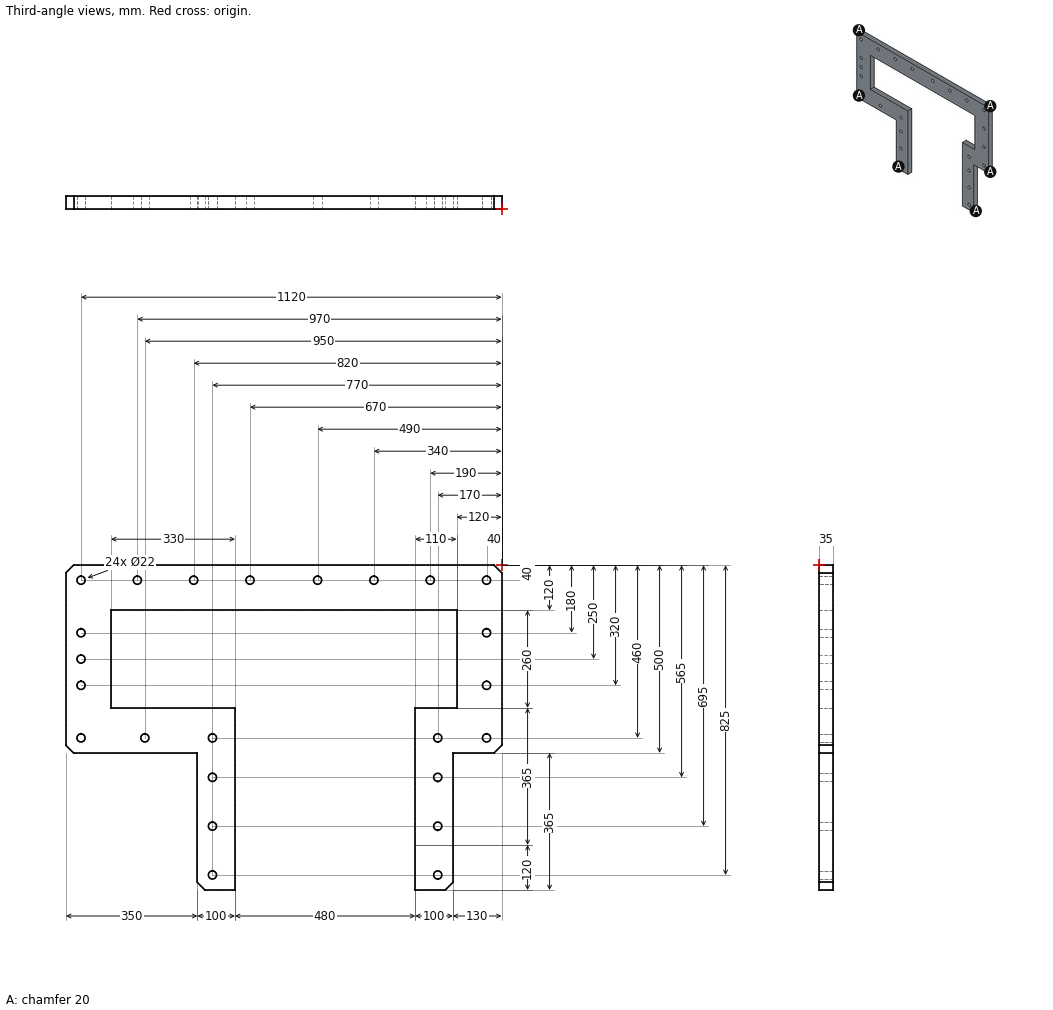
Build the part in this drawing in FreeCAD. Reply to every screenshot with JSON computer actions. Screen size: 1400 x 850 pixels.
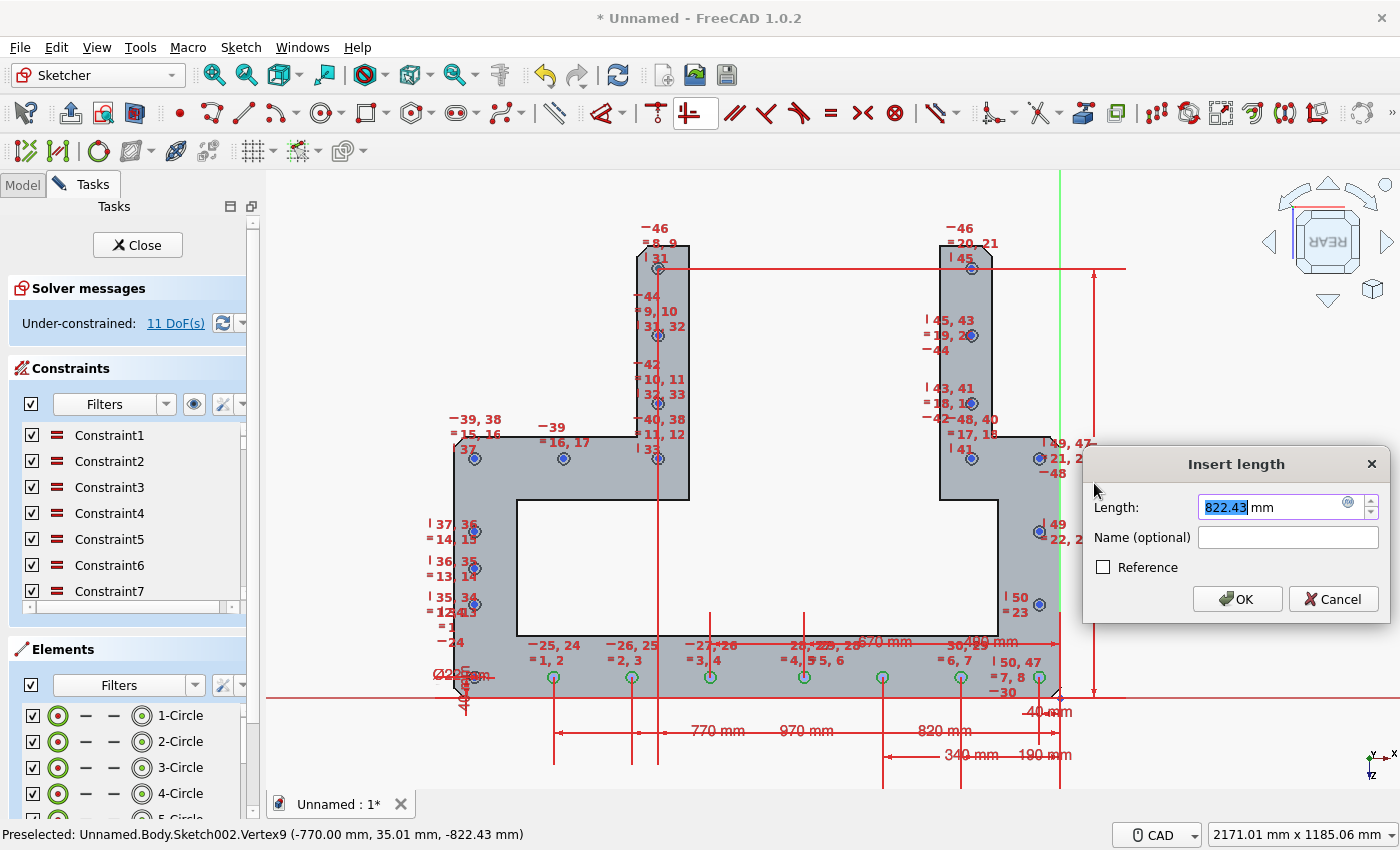
{"action": "type", "text": "825"}
{"action": "key", "text": "Return"}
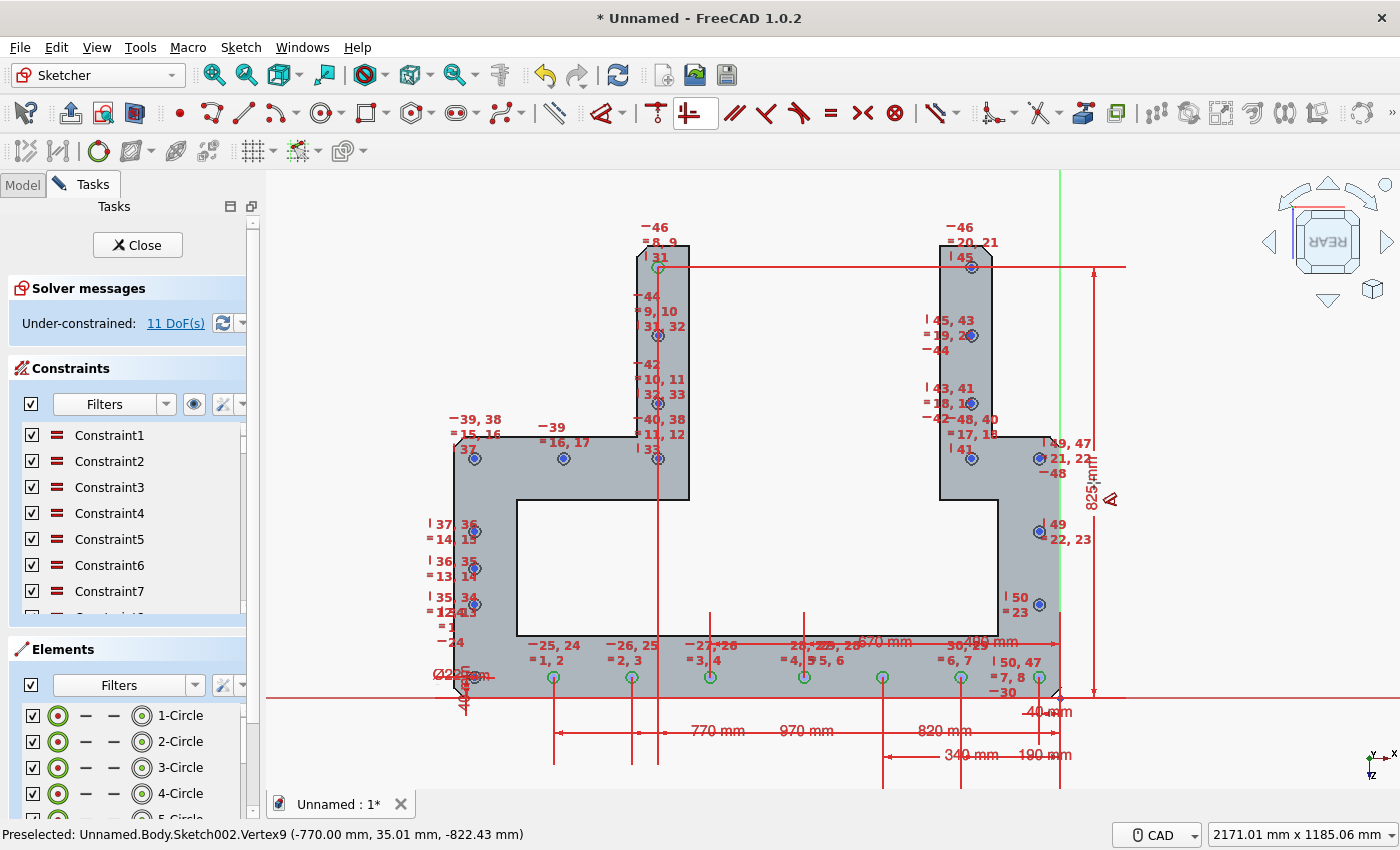
{"action": "left_click", "coordinate": [658, 336]}
{"action": "left_click", "coordinate": [1094, 517]}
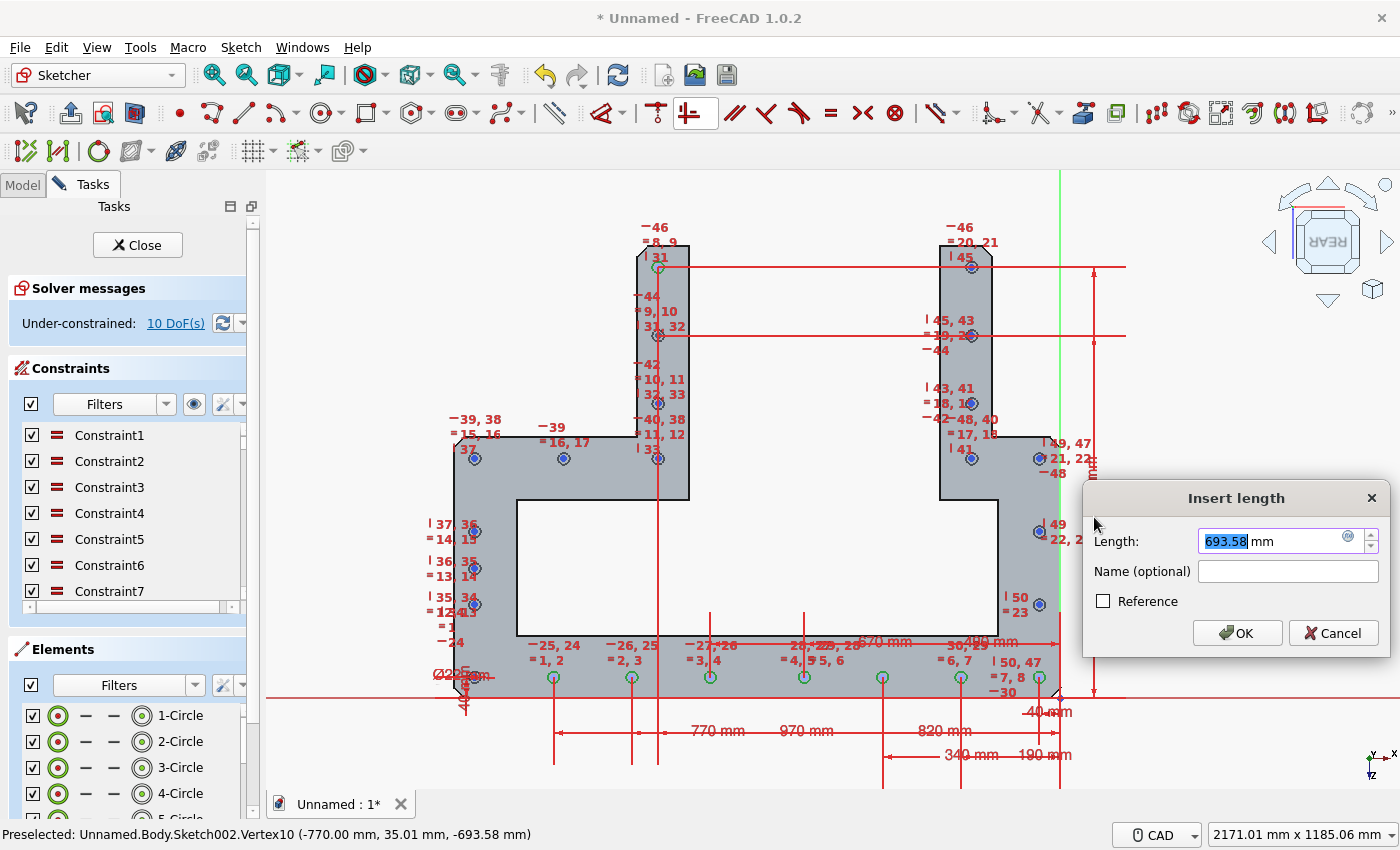
{"action": "type", "text": "695"}
{"action": "key", "text": "Return"}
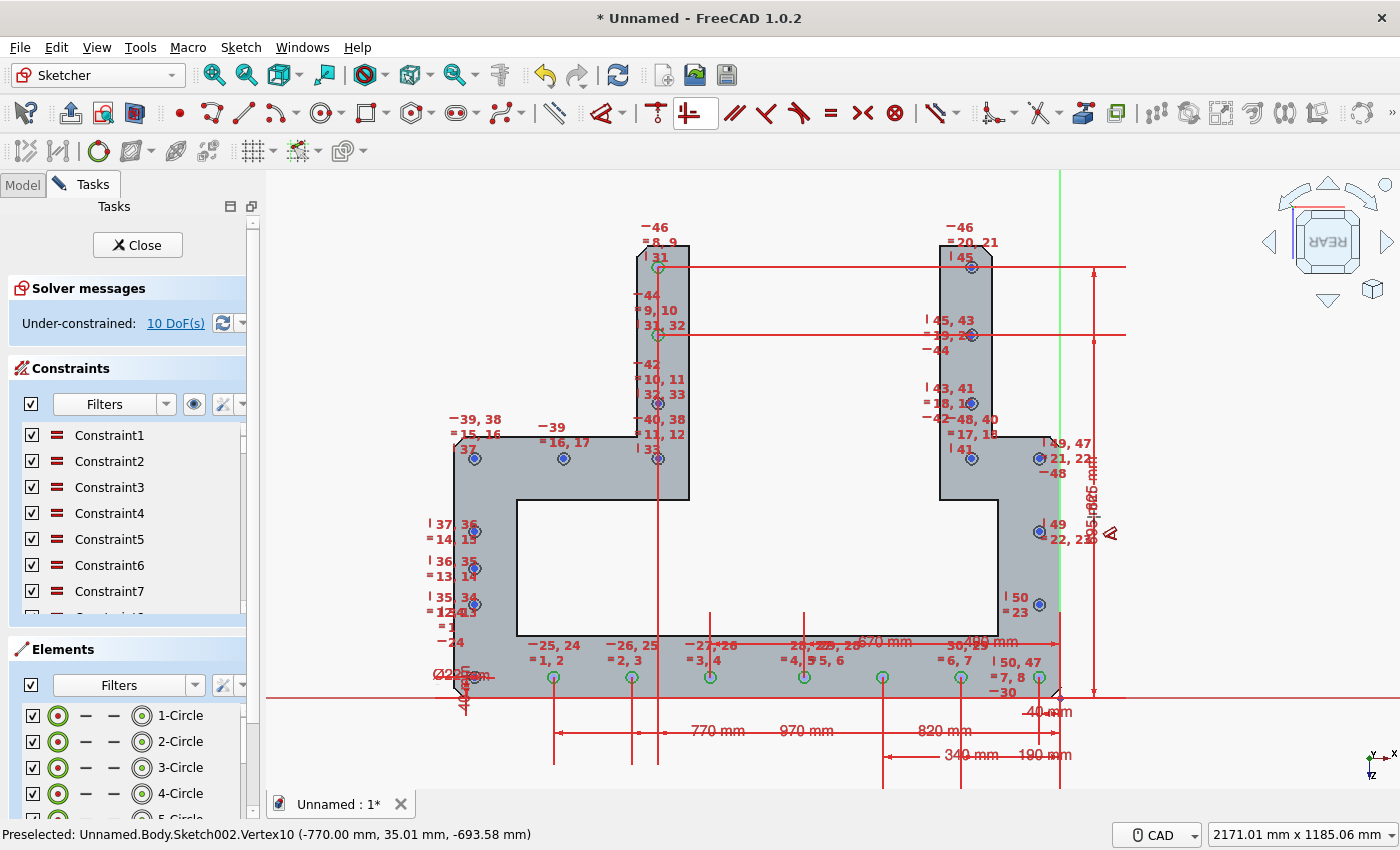
{"action": "left_click", "coordinate": [658, 404]}
{"action": "left_click", "coordinate": [1094, 551]}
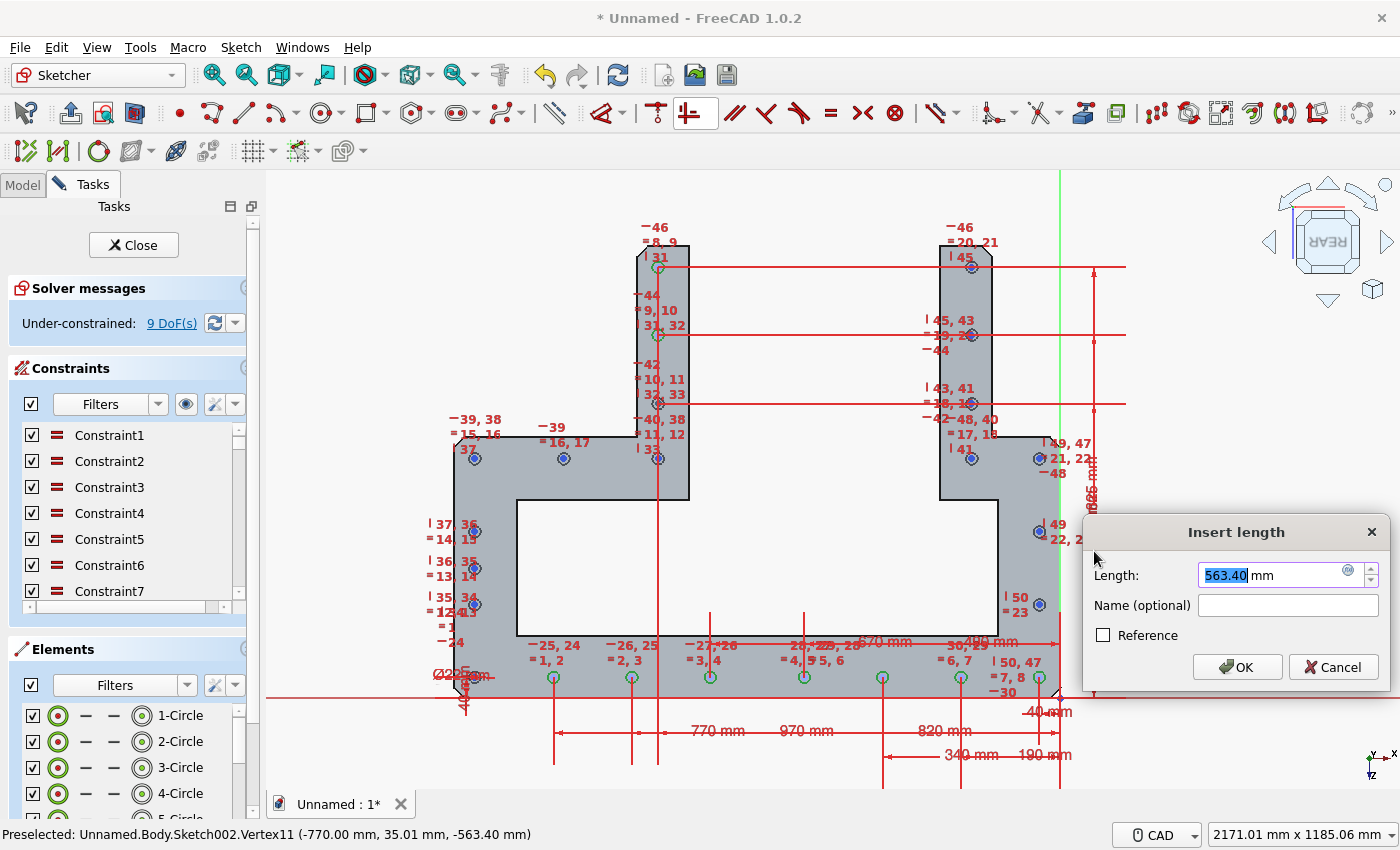
{"action": "type", "text": "565"}
{"action": "key", "text": "Return"}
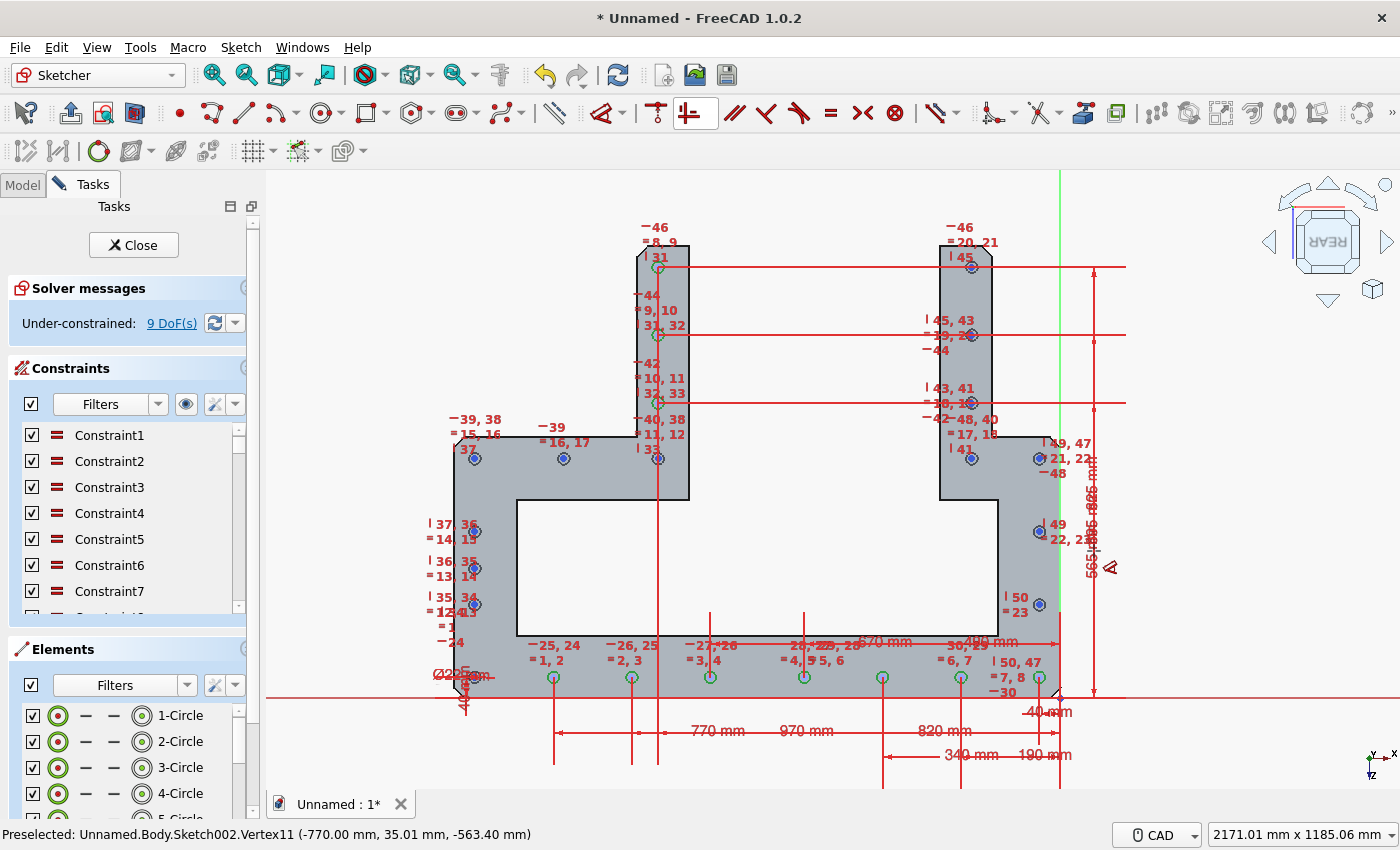
{"action": "left_click", "coordinate": [658, 459]}
{"action": "left_click", "coordinate": [1094, 579]}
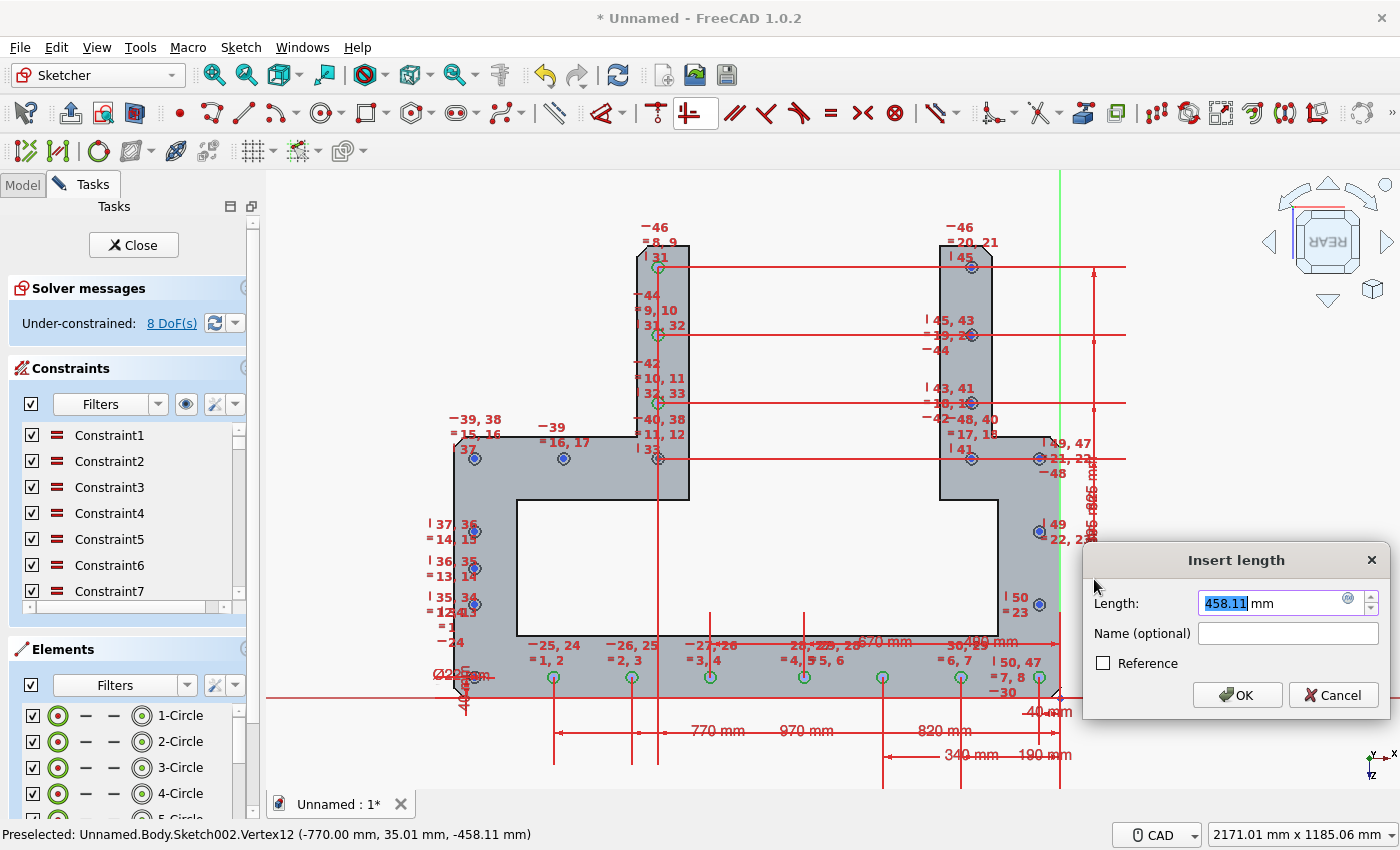
{"action": "type", "text": "460"}
{"action": "key", "text": "Return"}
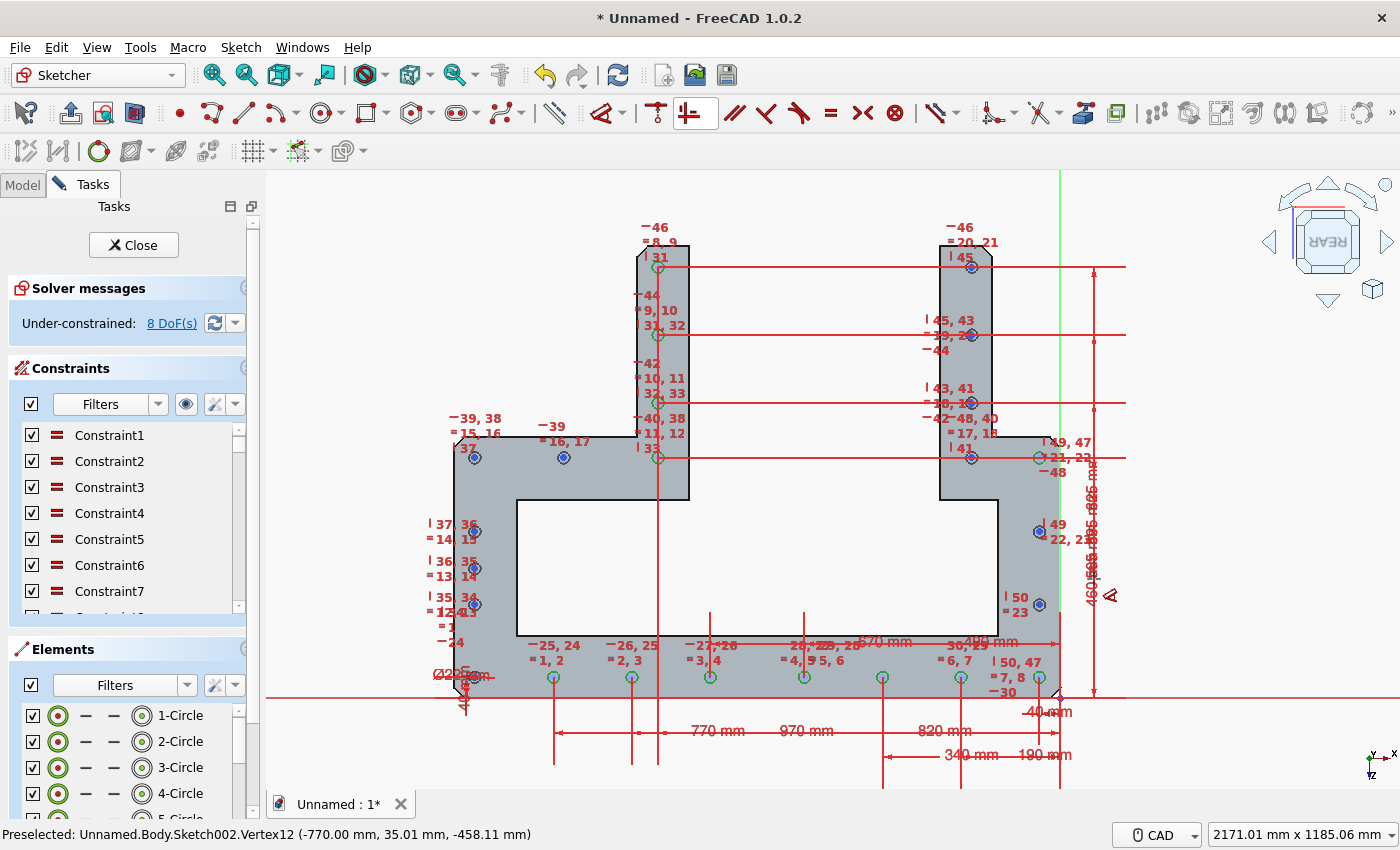
{"action": "left_click", "coordinate": [475, 605]}
{"action": "left_click", "coordinate": [1094, 652]}